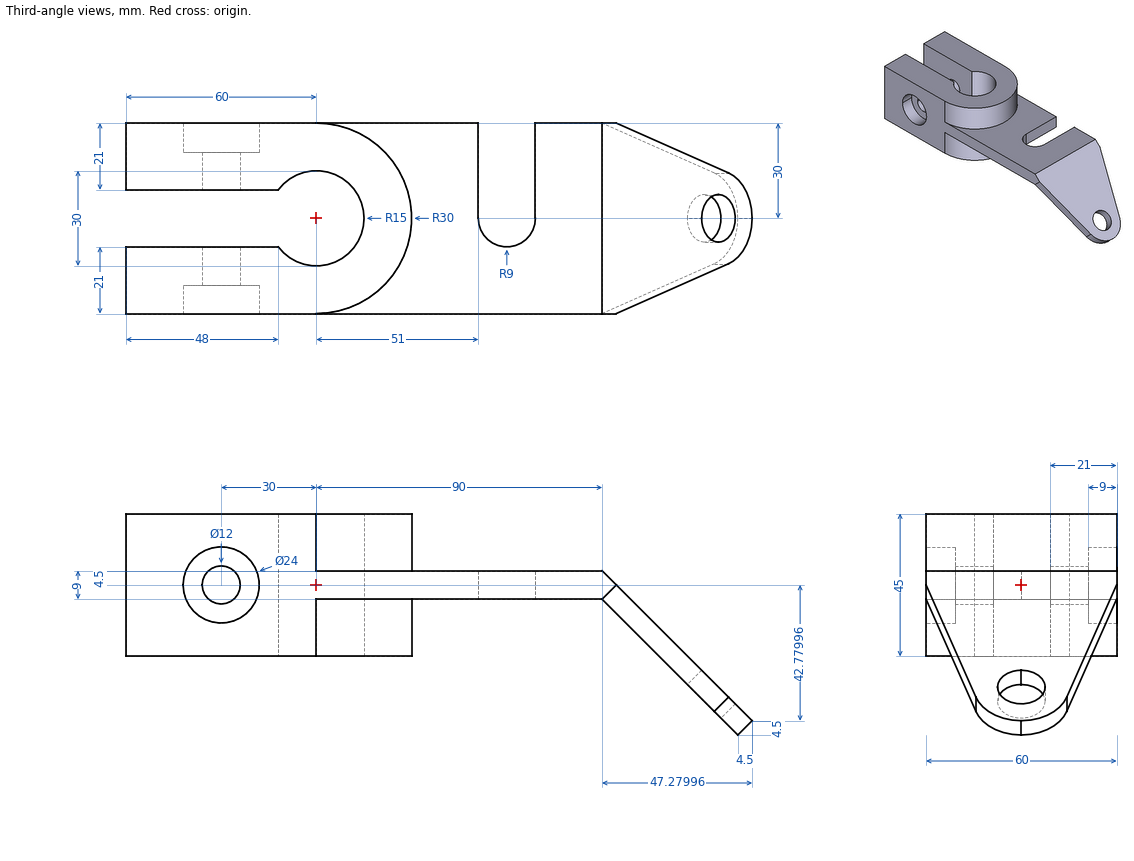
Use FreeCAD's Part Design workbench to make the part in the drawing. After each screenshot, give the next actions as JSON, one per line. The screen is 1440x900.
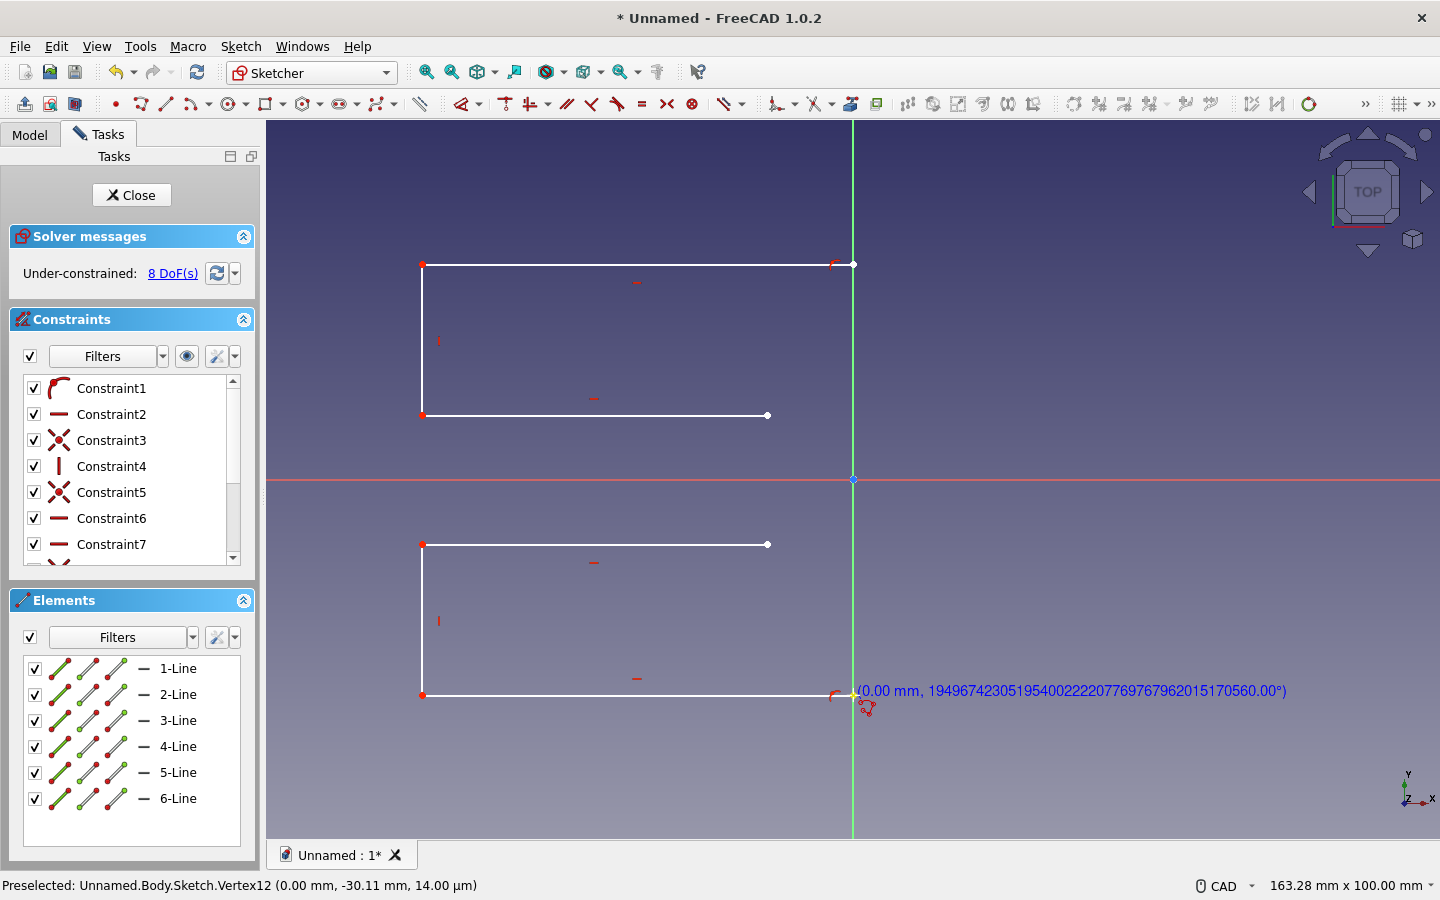
{"action": "left_click", "coordinate": [208, 104]}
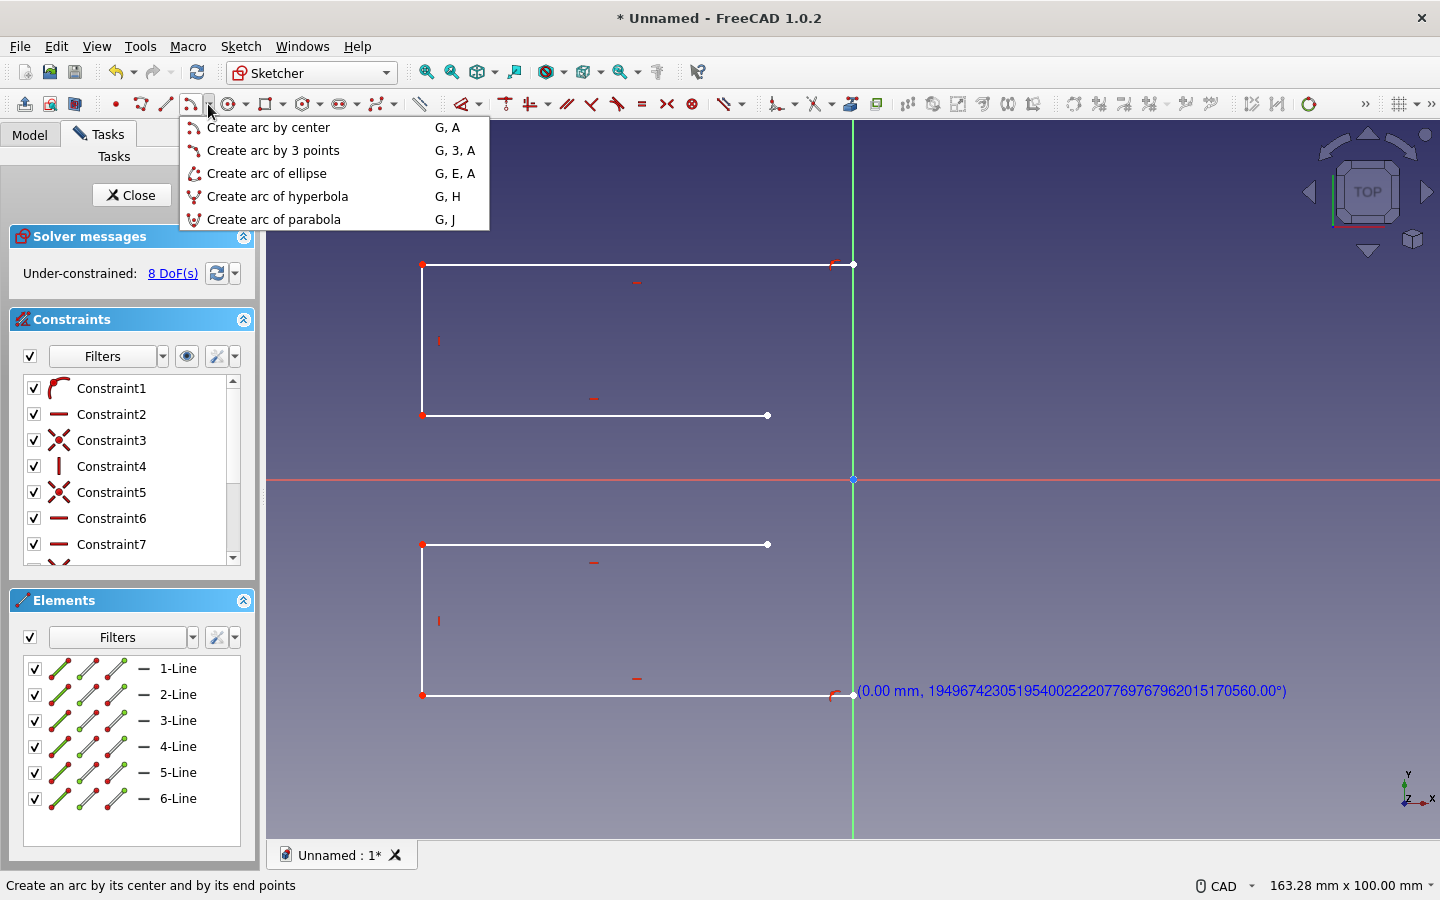
{"action": "left_click", "coordinate": [334, 150]}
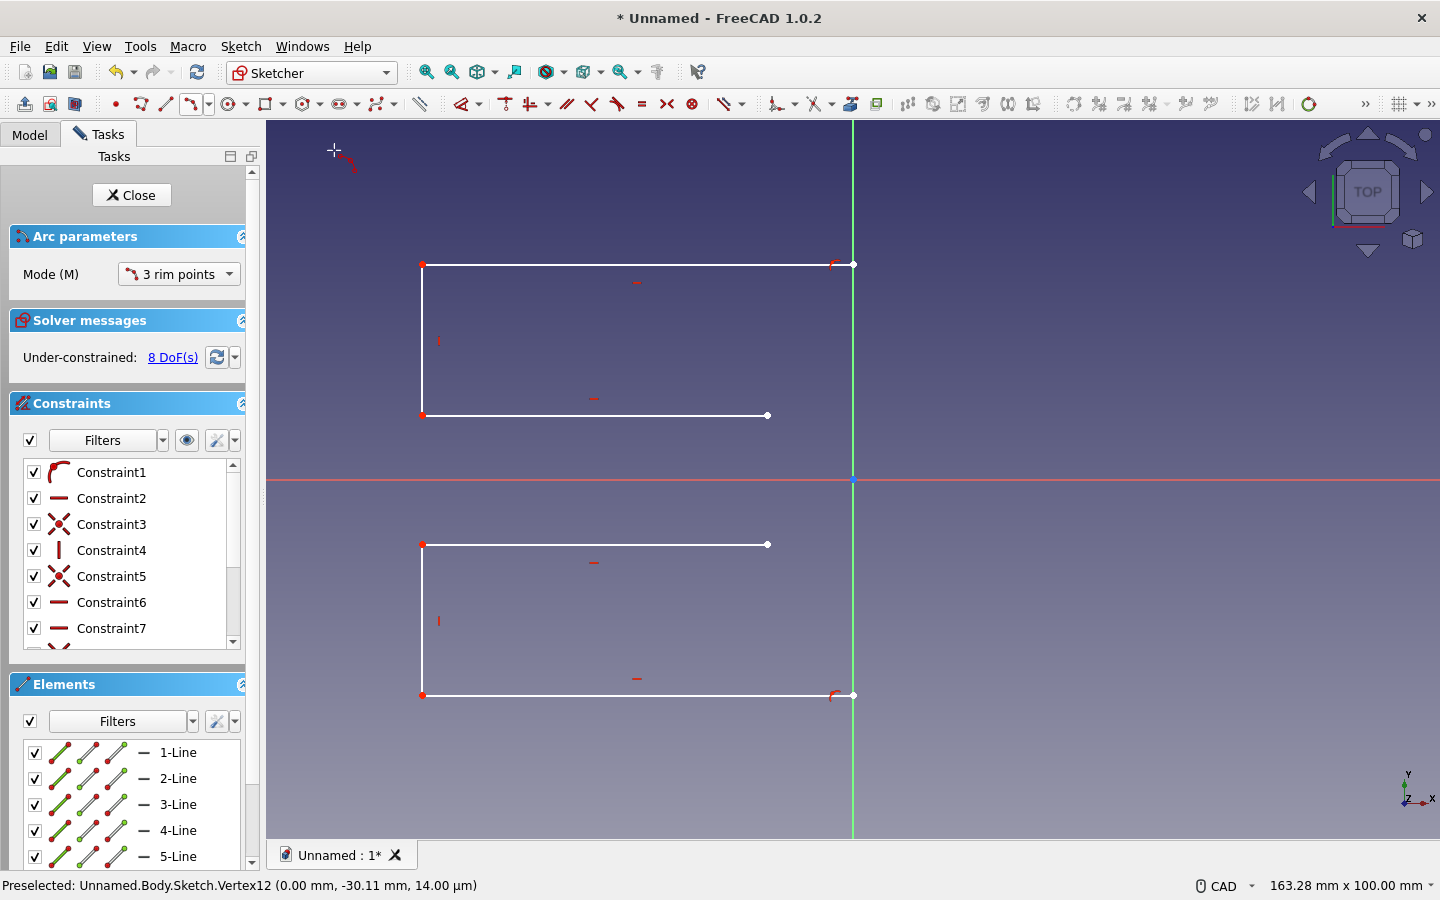
{"action": "left_click", "coordinate": [767, 416]}
{"action": "left_click", "coordinate": [767, 545]}
{"action": "left_click", "coordinate": [948, 531]}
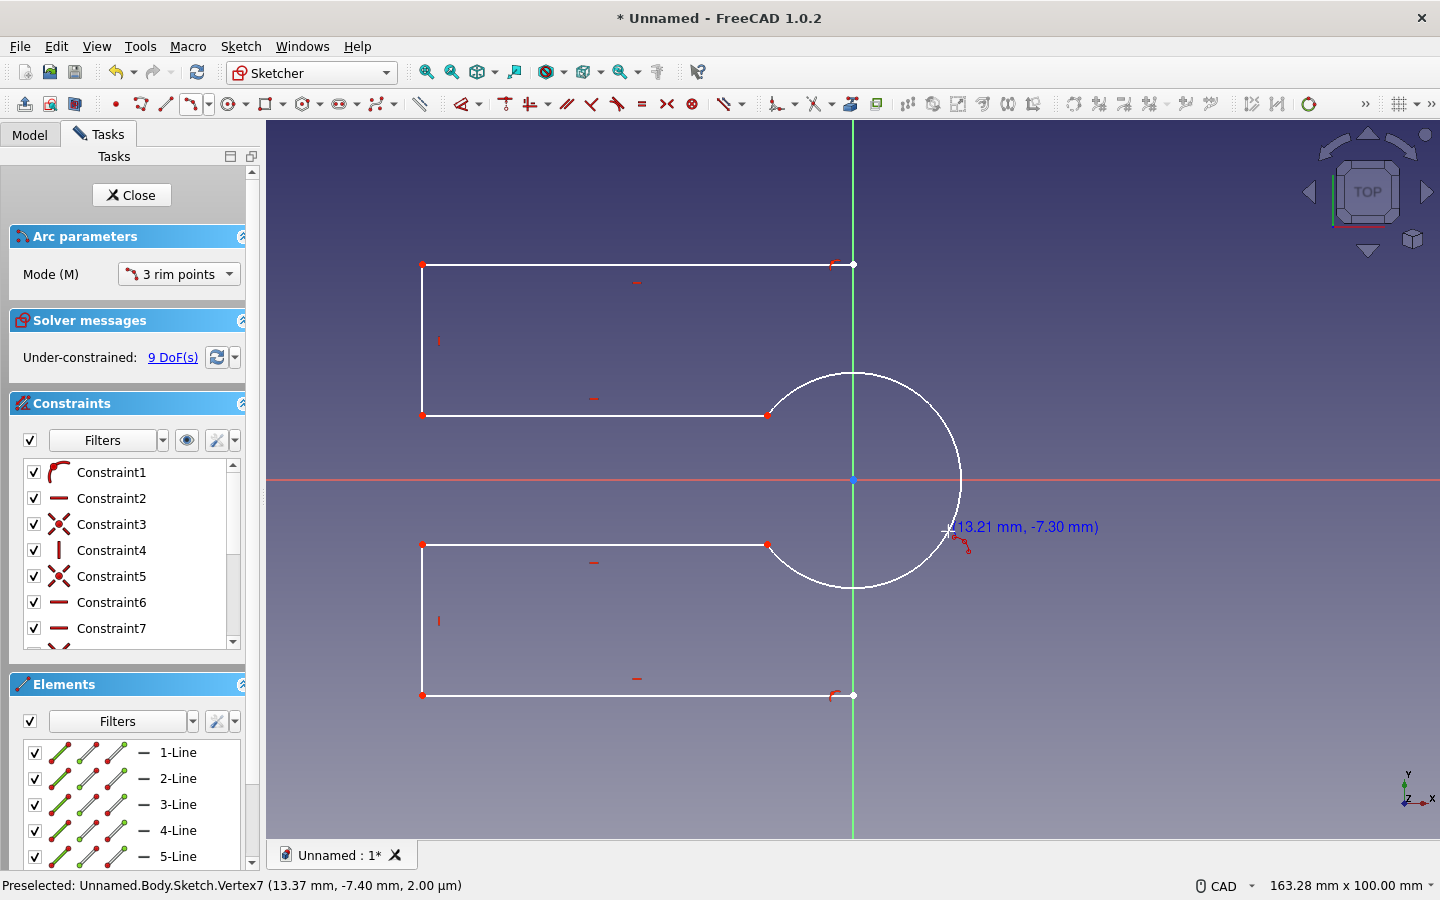
{"action": "left_click", "coordinate": [853, 696]}
{"action": "left_click", "coordinate": [853, 265]}
{"action": "left_click", "coordinate": [1058, 546]}
{"action": "key", "text": "Escape"}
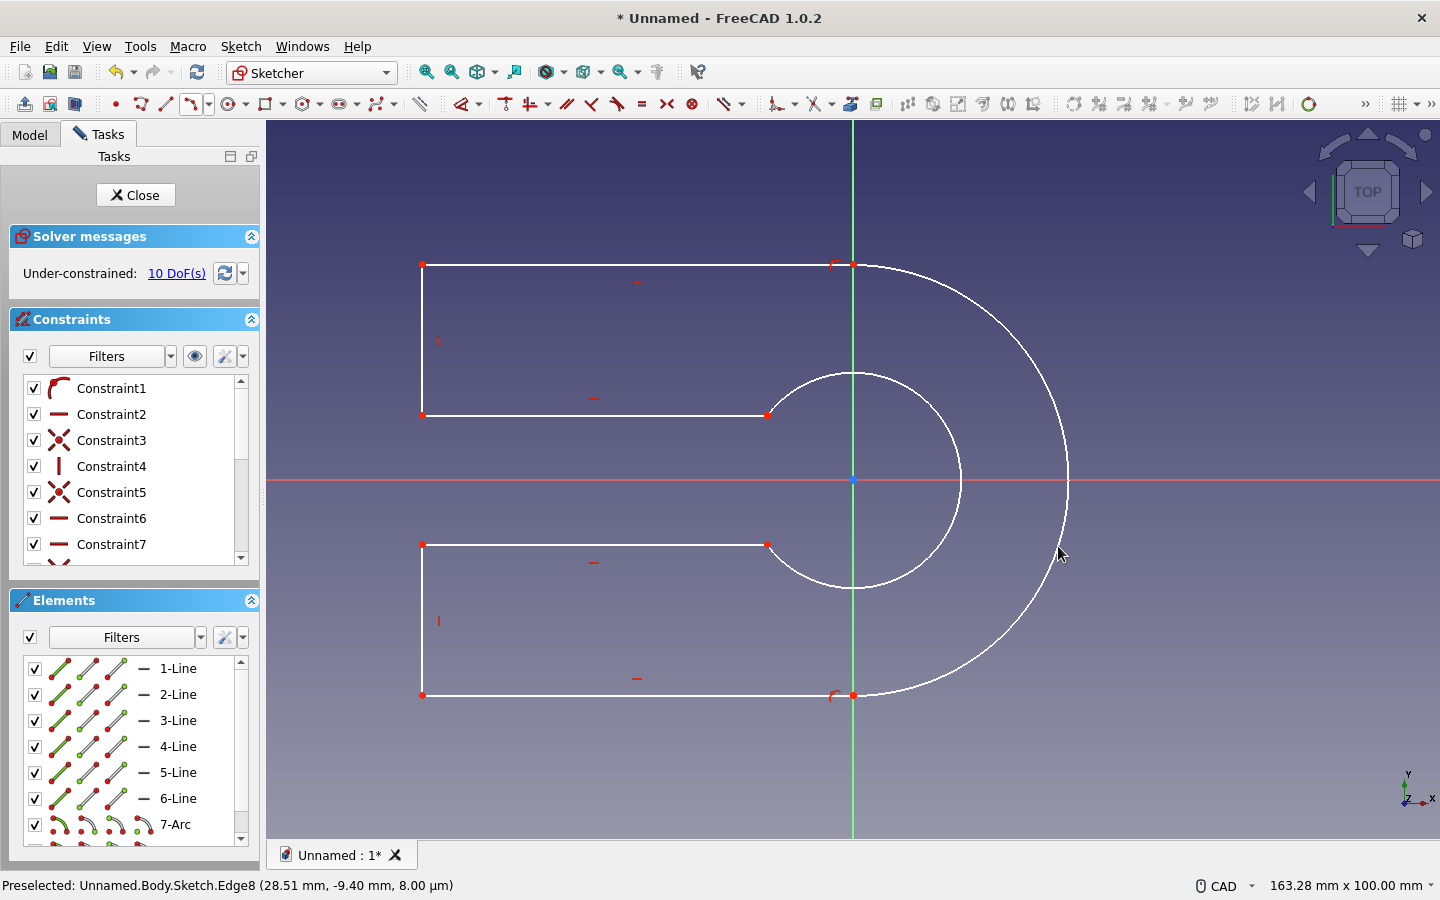
{"action": "left_click", "coordinate": [912, 571]}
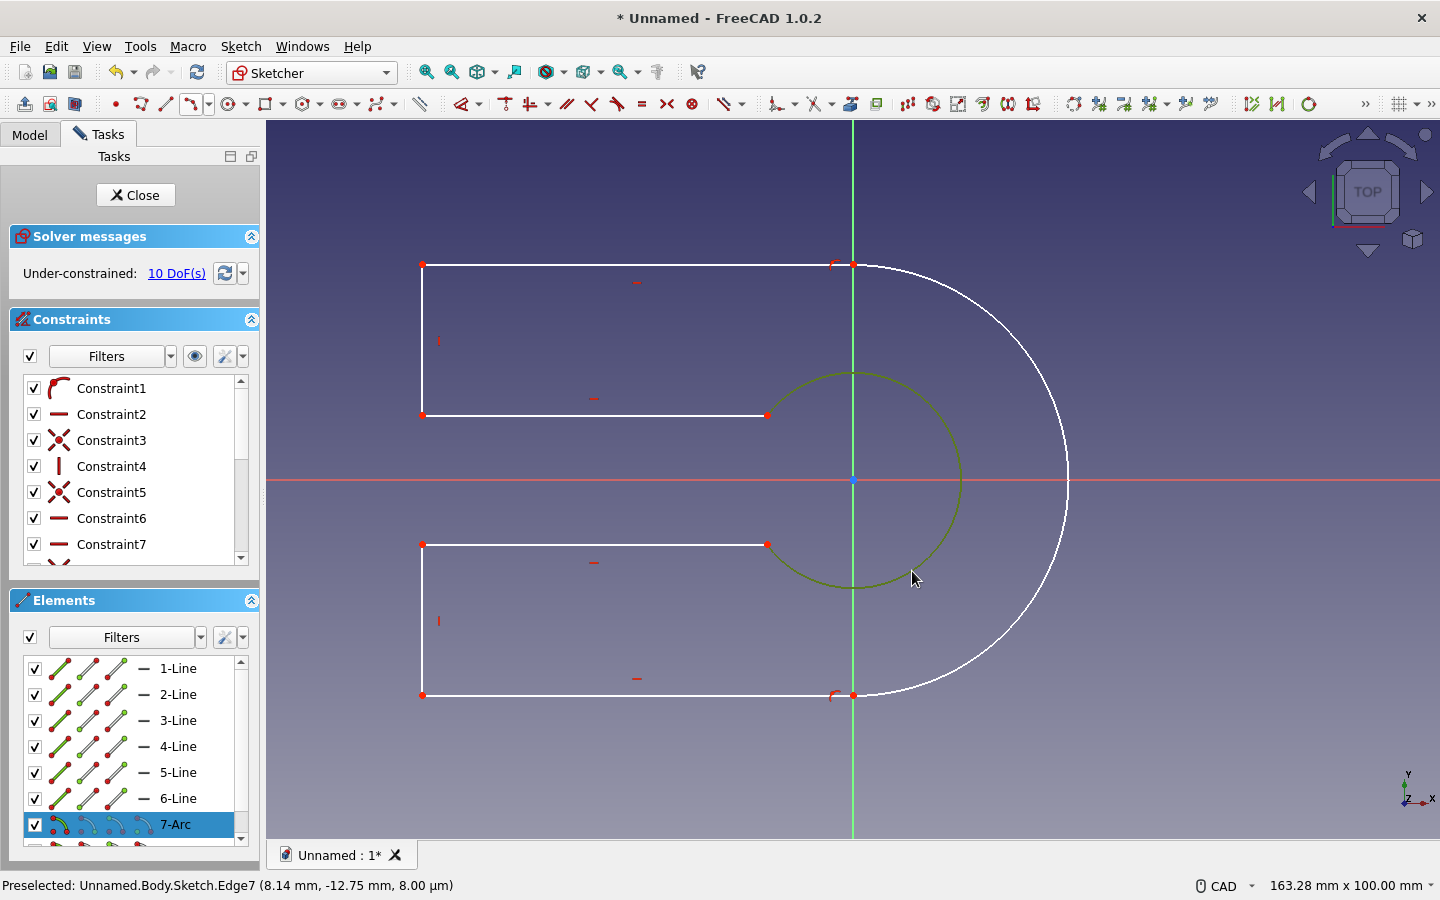
{"action": "left_click", "coordinate": [1027, 607]}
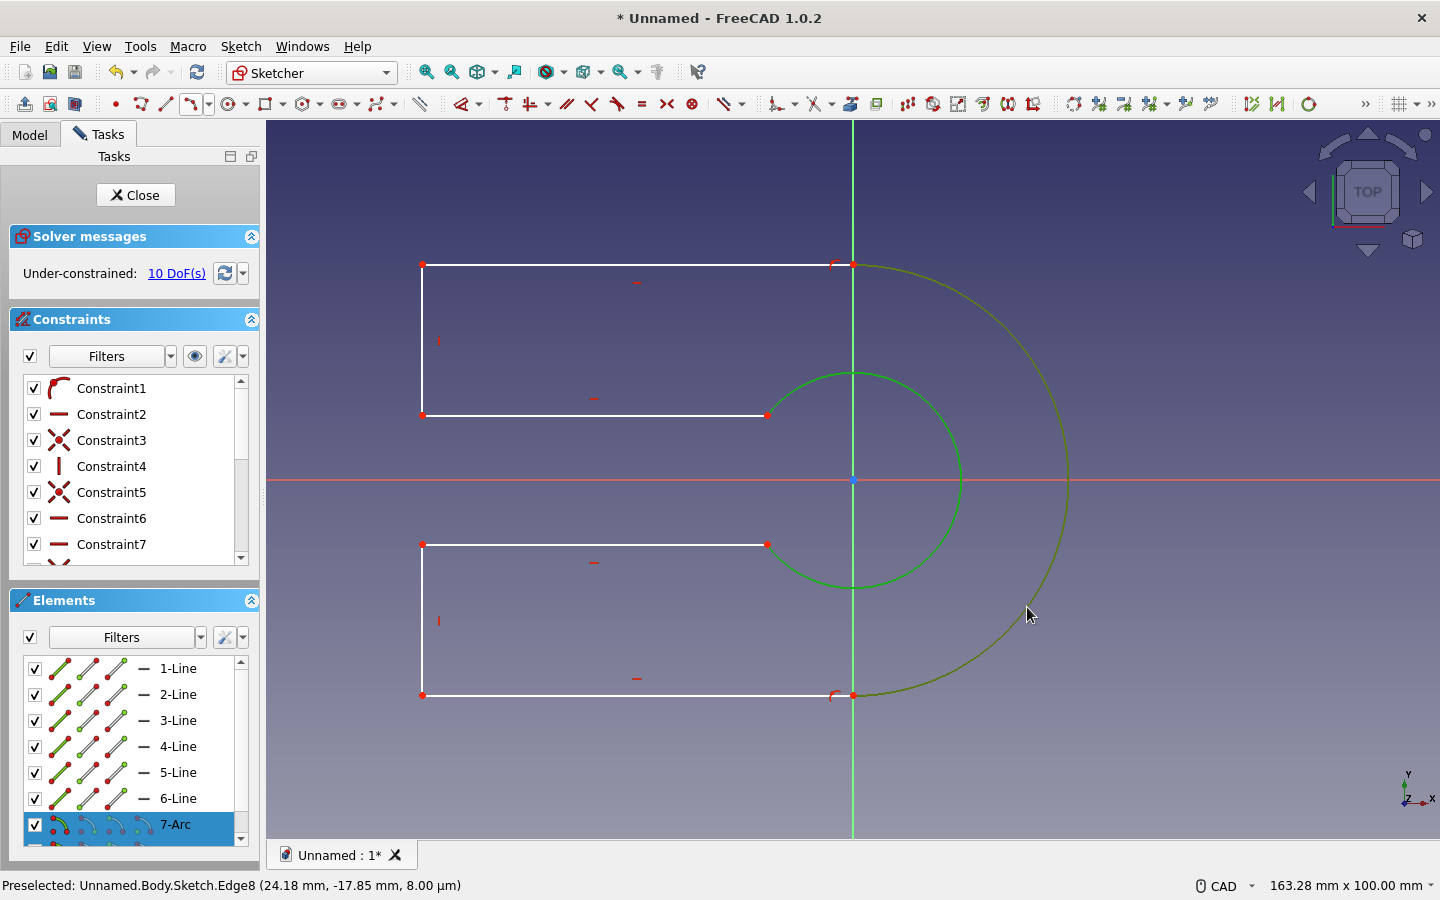
{"action": "left_click", "coordinate": [505, 104]}